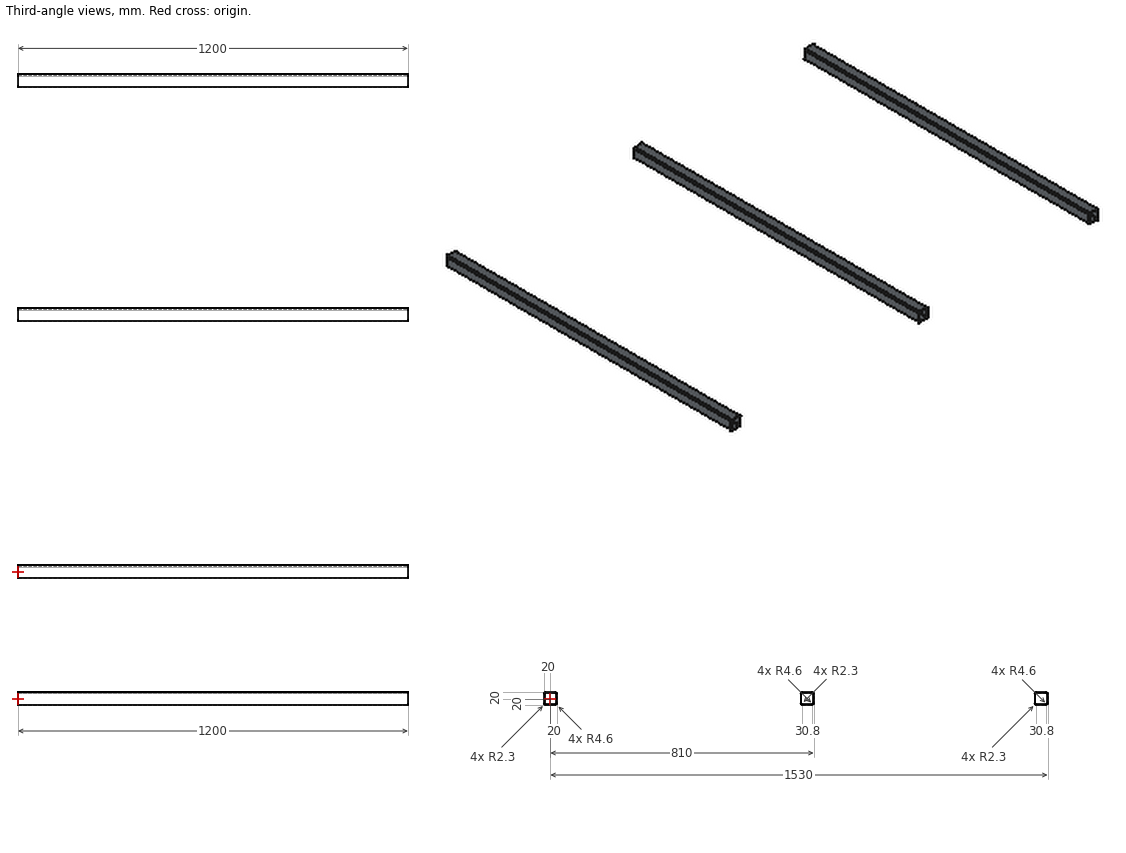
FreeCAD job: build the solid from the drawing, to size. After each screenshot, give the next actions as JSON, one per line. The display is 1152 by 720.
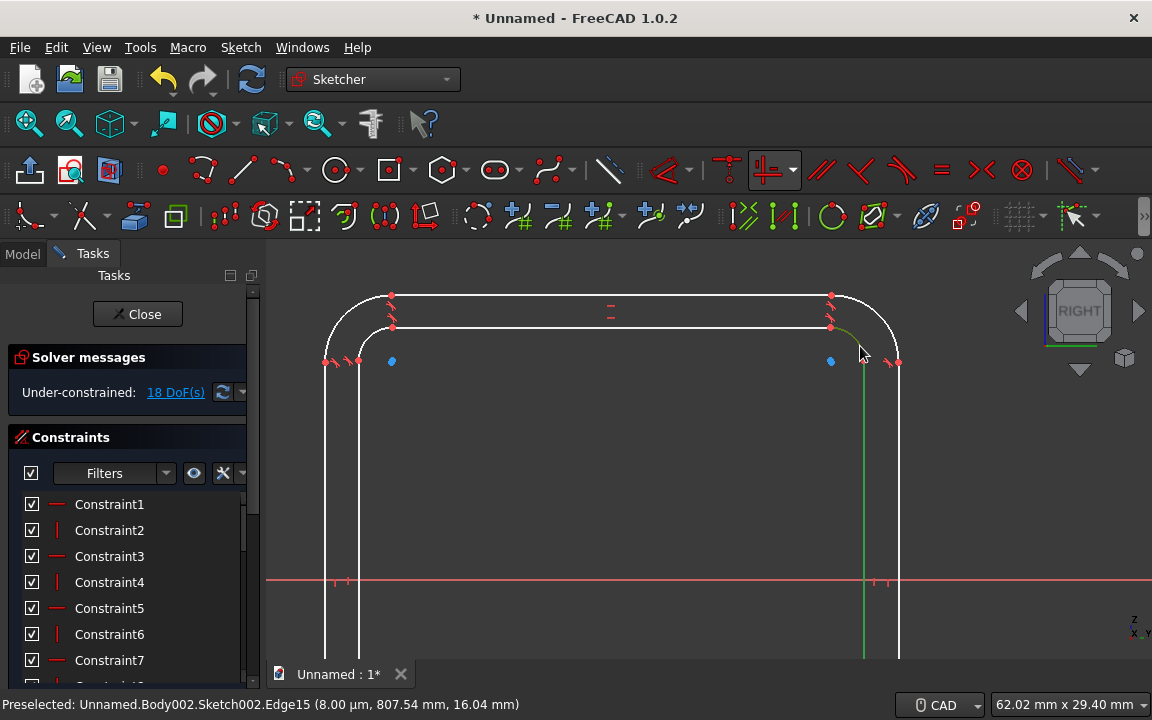
{"action": "key", "text": "t"}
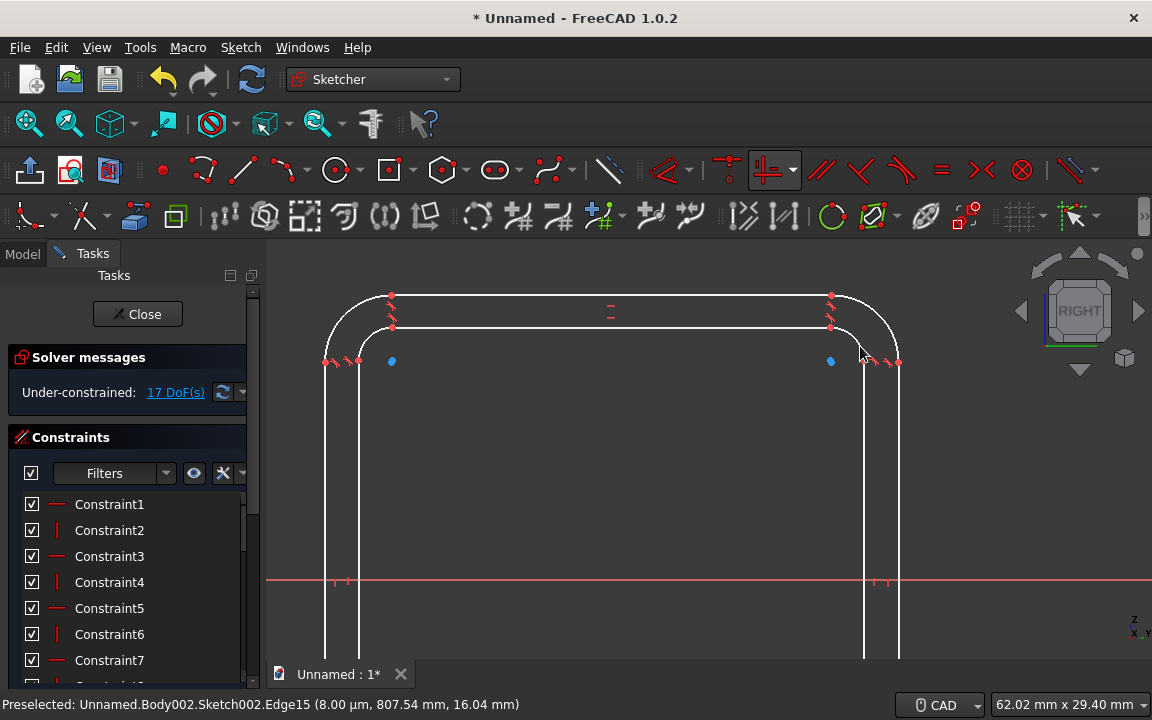
{"action": "left_click", "coordinate": [864, 493]}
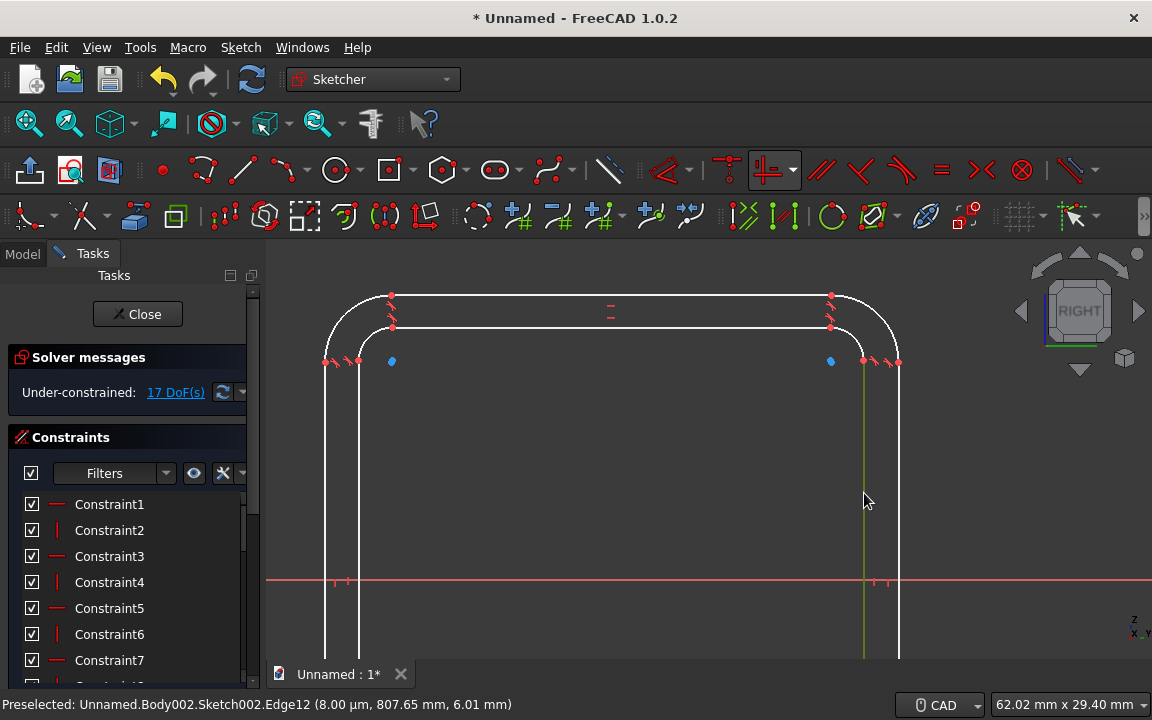
{"action": "scroll", "coordinate": [664, 342], "scroll_direction": "down", "scroll_amount": 4}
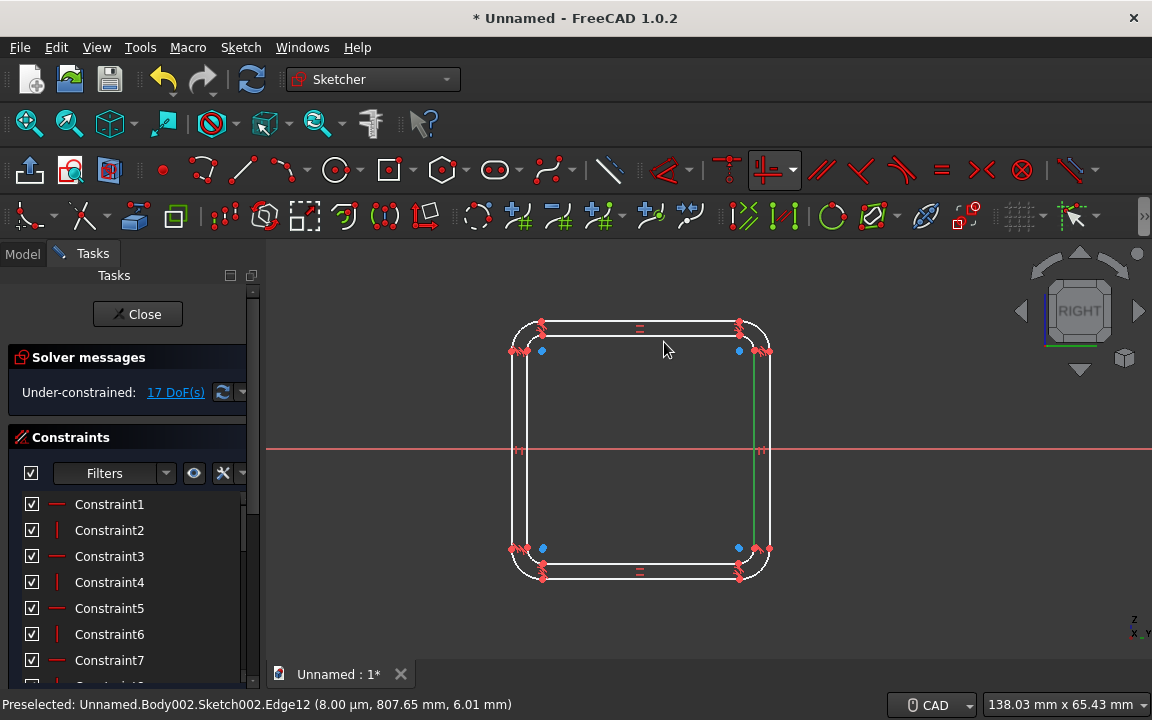
{"action": "scroll", "coordinate": [745, 562], "scroll_direction": "up", "scroll_amount": 4}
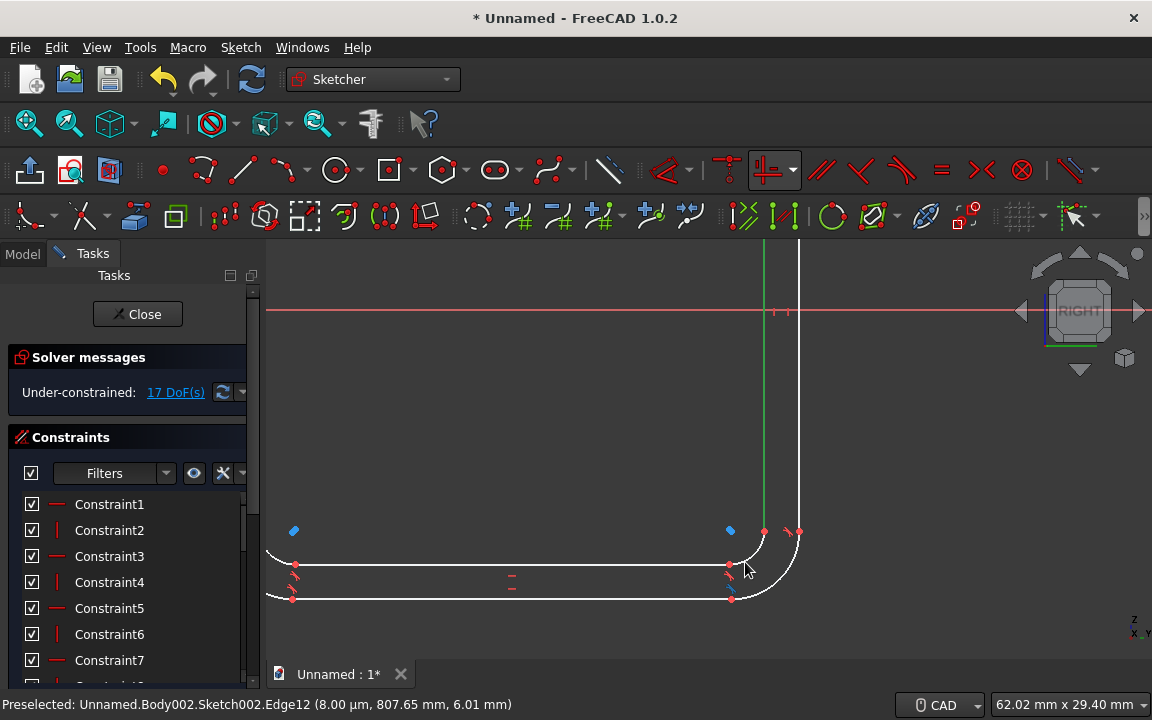
{"action": "left_click", "coordinate": [745, 561]}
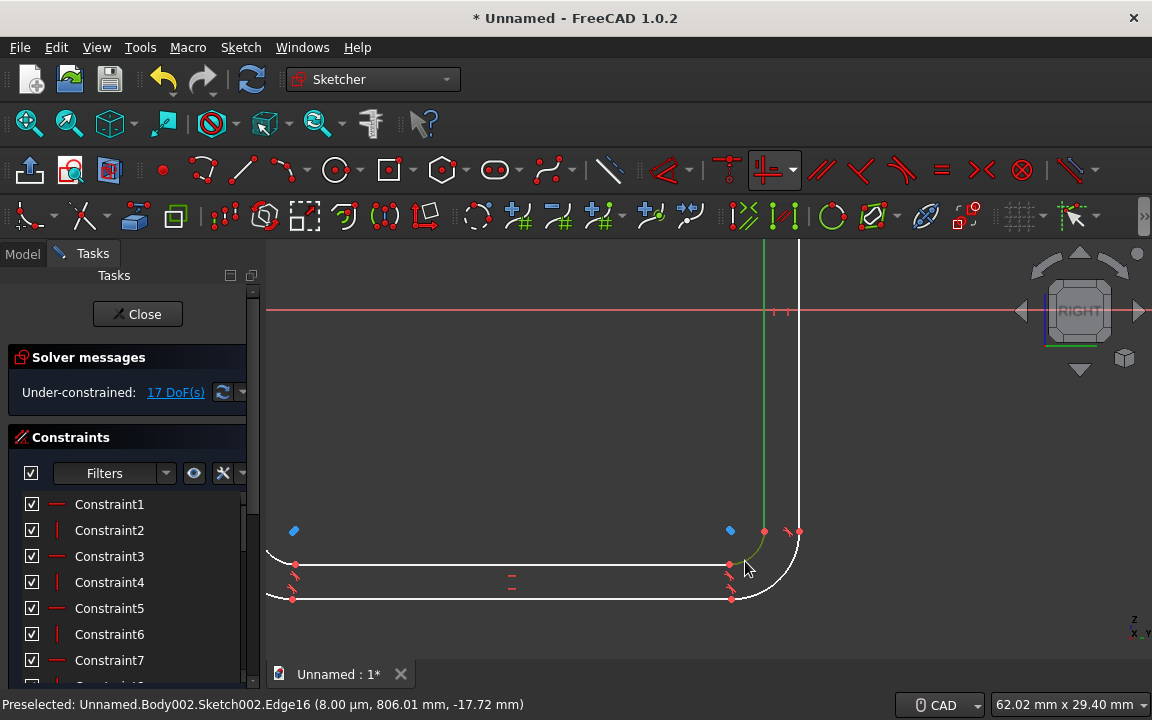
{"action": "left_click", "coordinate": [902, 170]}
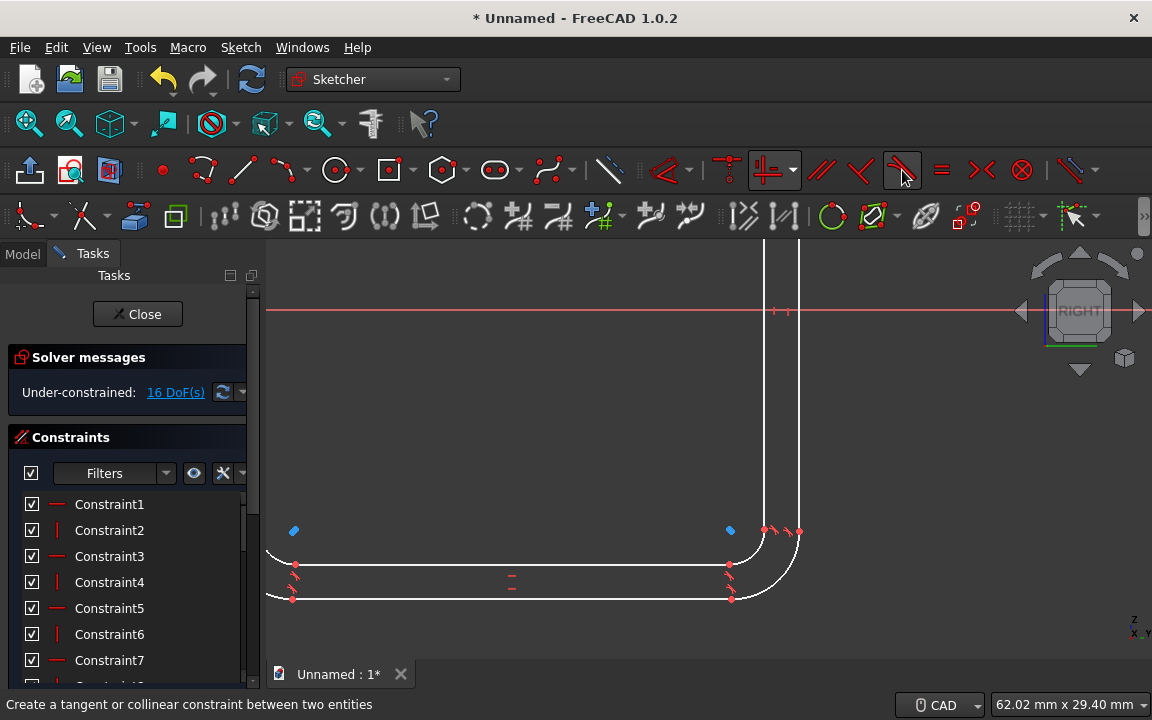
{"action": "scroll", "coordinate": [745, 563], "scroll_direction": "down", "scroll_amount": 4}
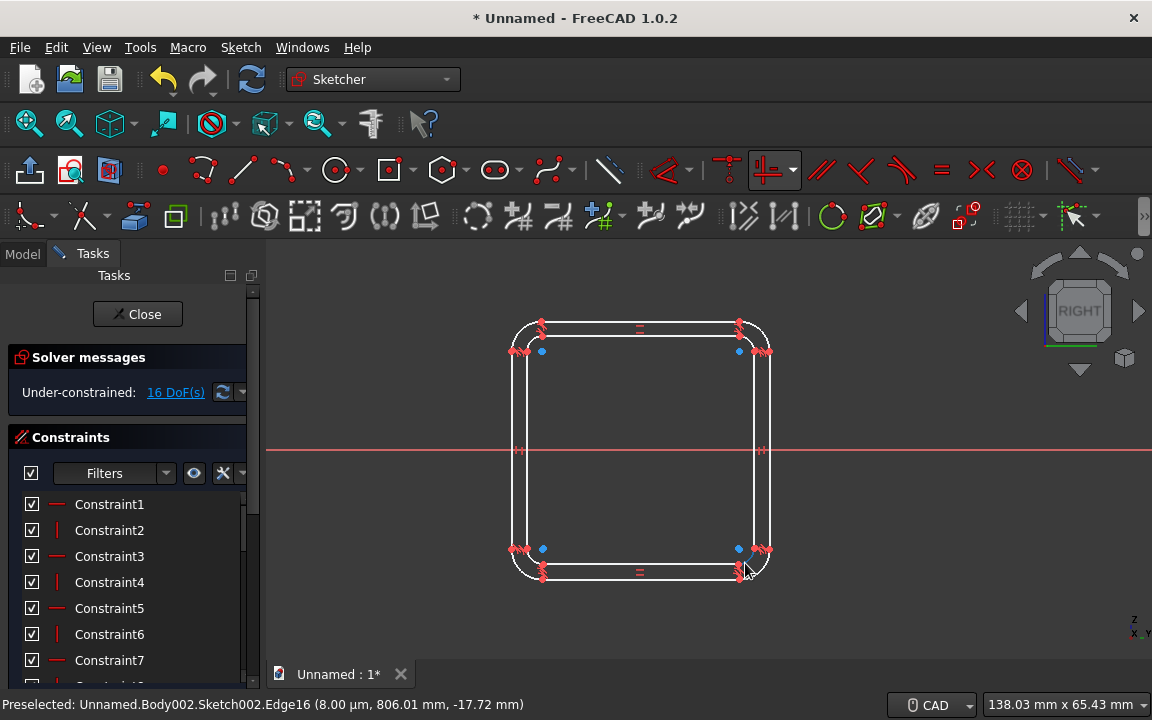
{"action": "left_click", "coordinate": [515, 563]}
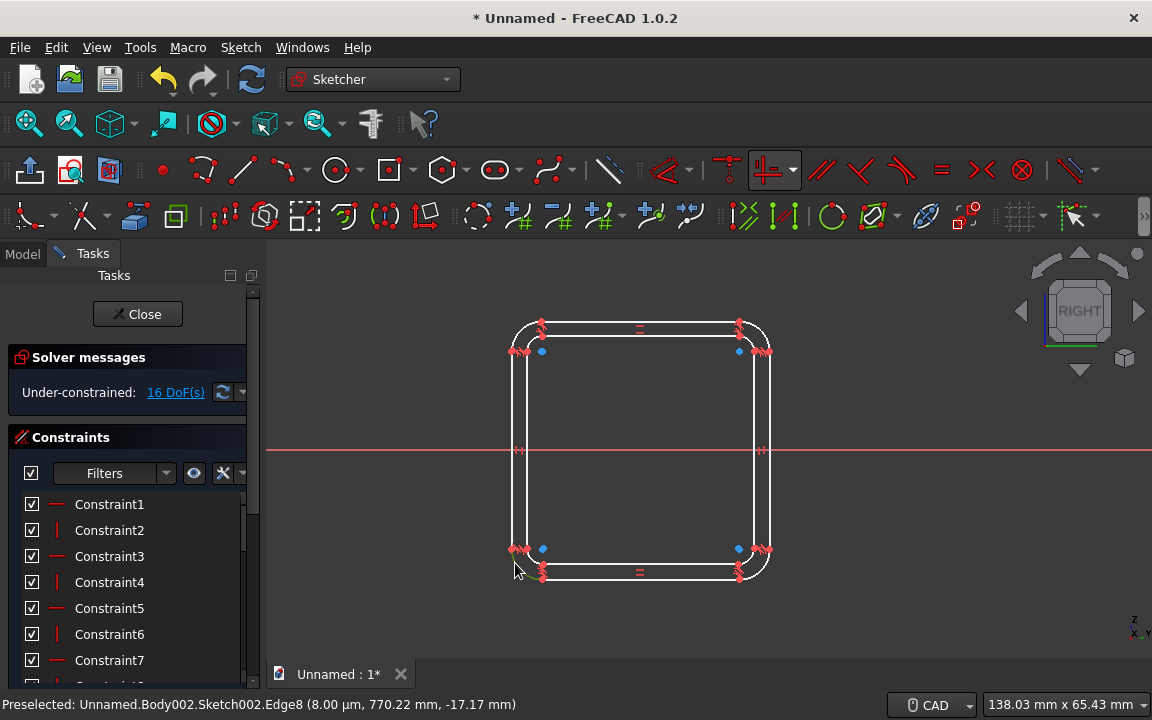
{"action": "left_click", "coordinate": [532, 559]}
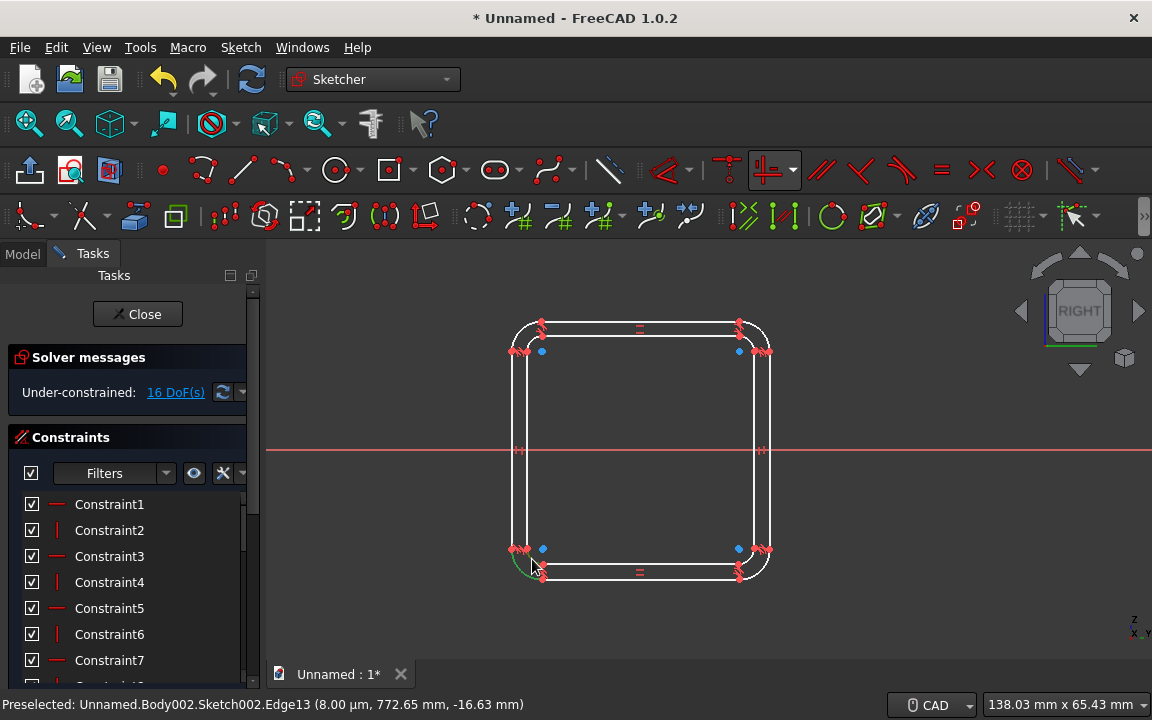
{"action": "key", "text": "c"}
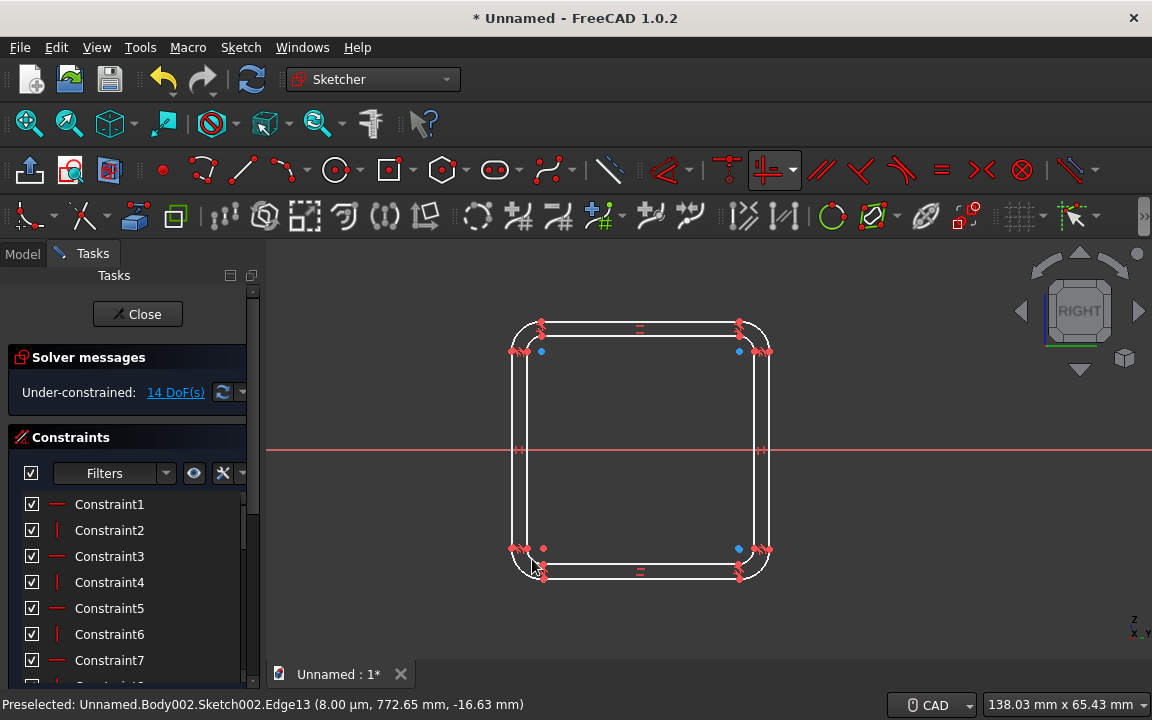
{"action": "left_click", "coordinate": [528, 325]}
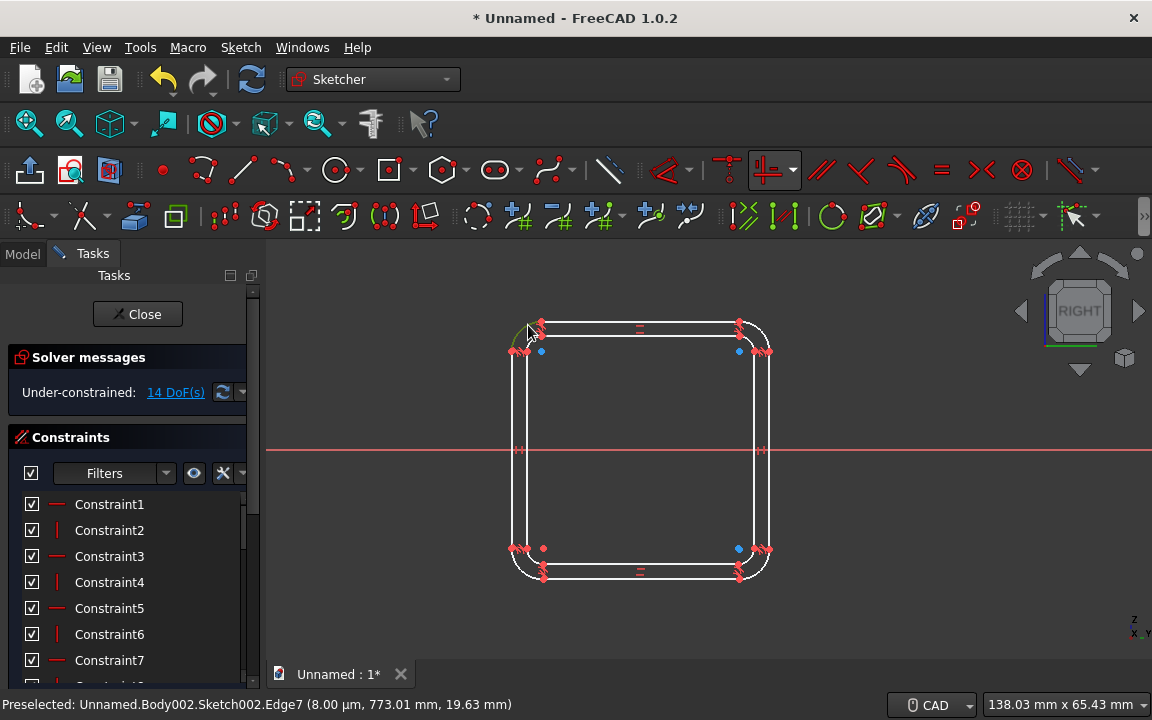
{"action": "left_click", "coordinate": [531, 341]}